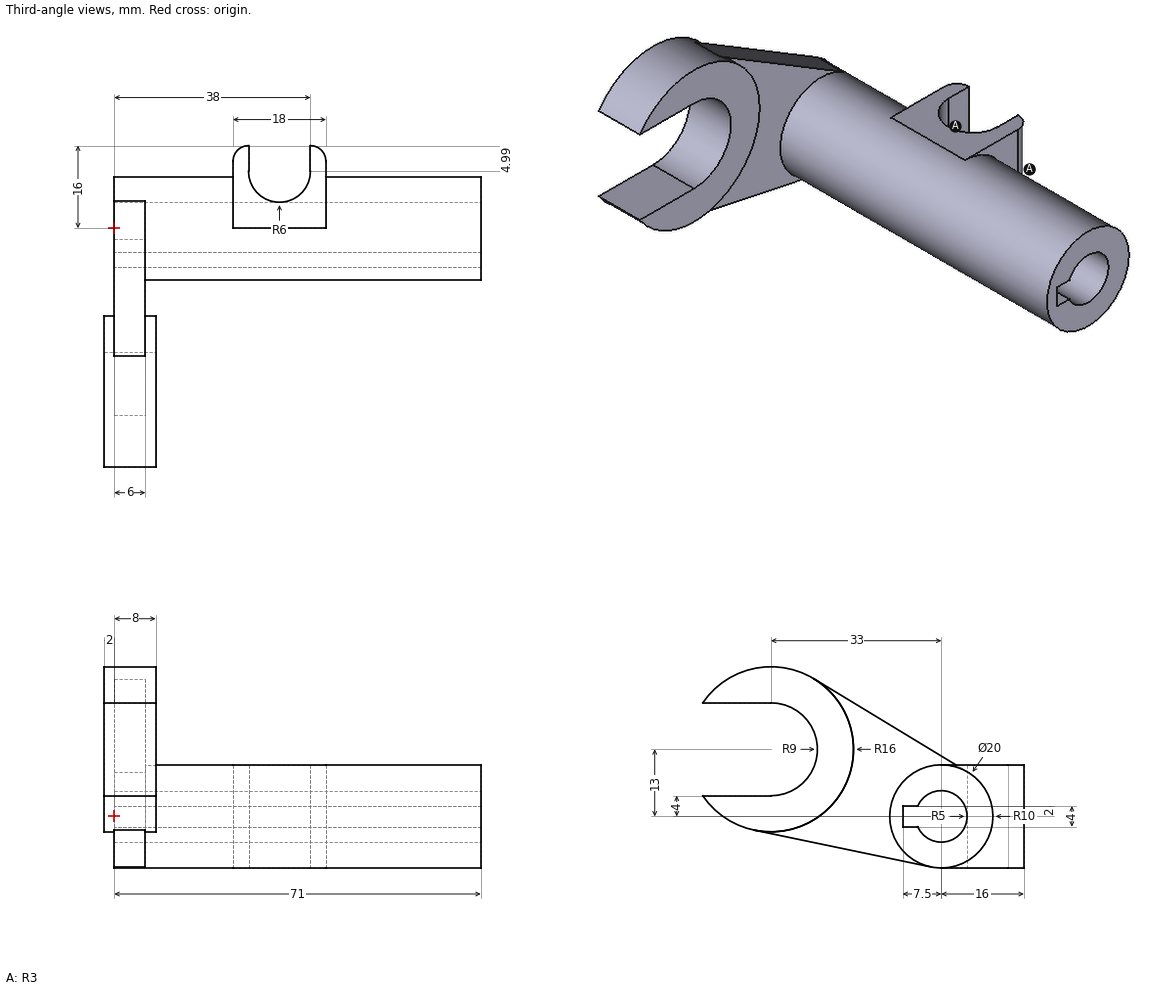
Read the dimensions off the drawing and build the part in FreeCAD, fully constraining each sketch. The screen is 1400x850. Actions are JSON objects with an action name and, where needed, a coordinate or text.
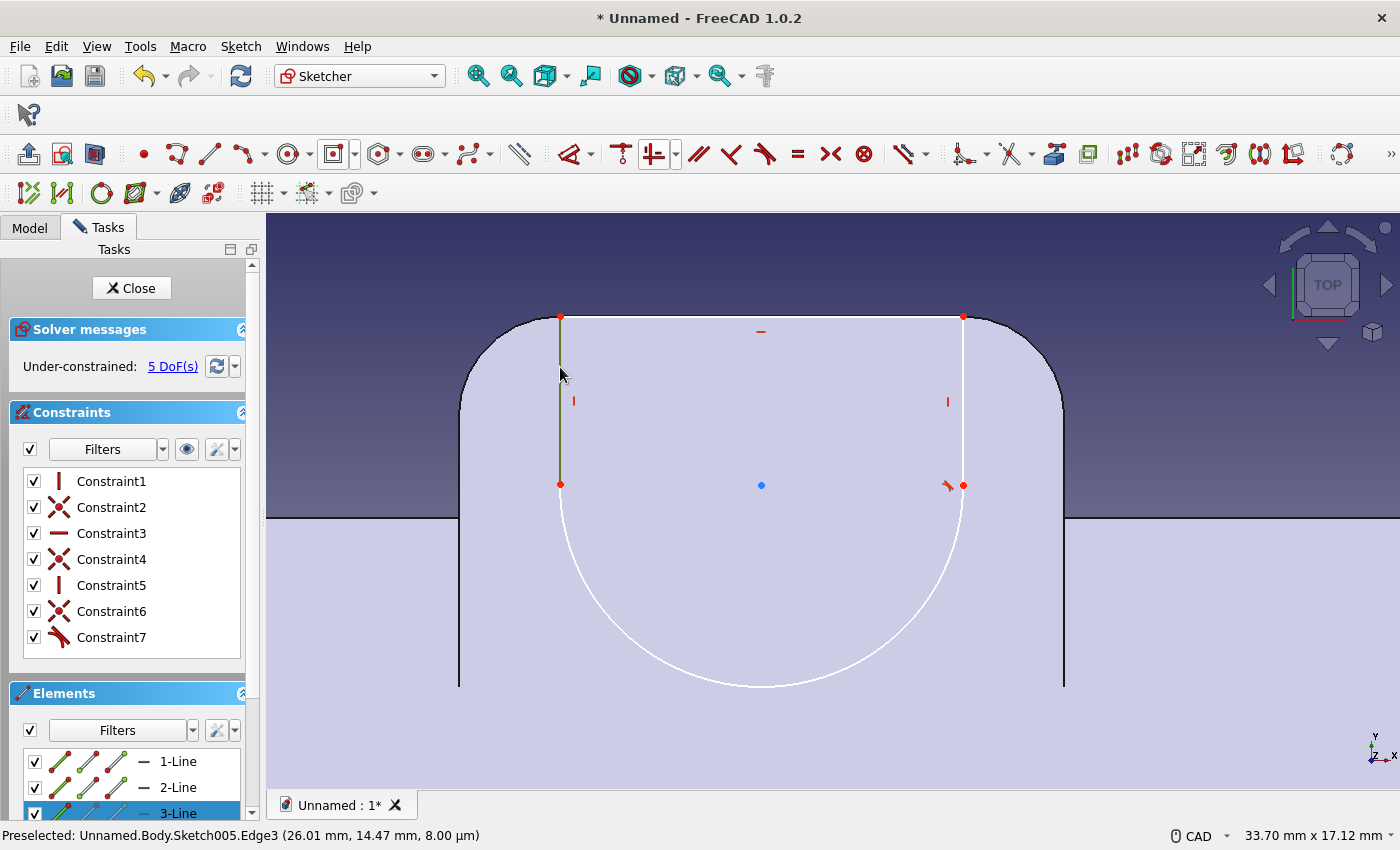
{"action": "left_click", "coordinate": [643, 648]}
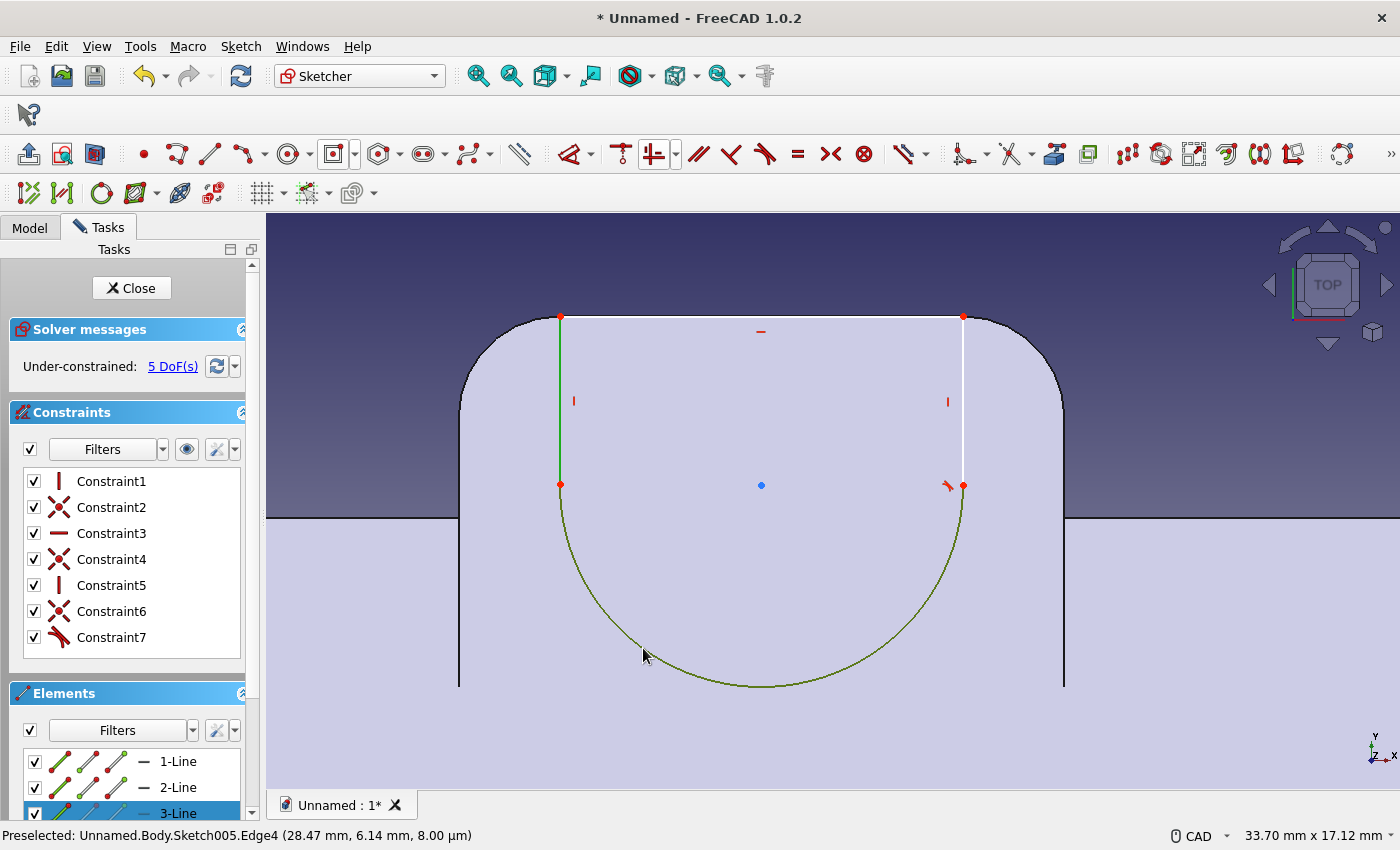
{"action": "key", "text": "t"}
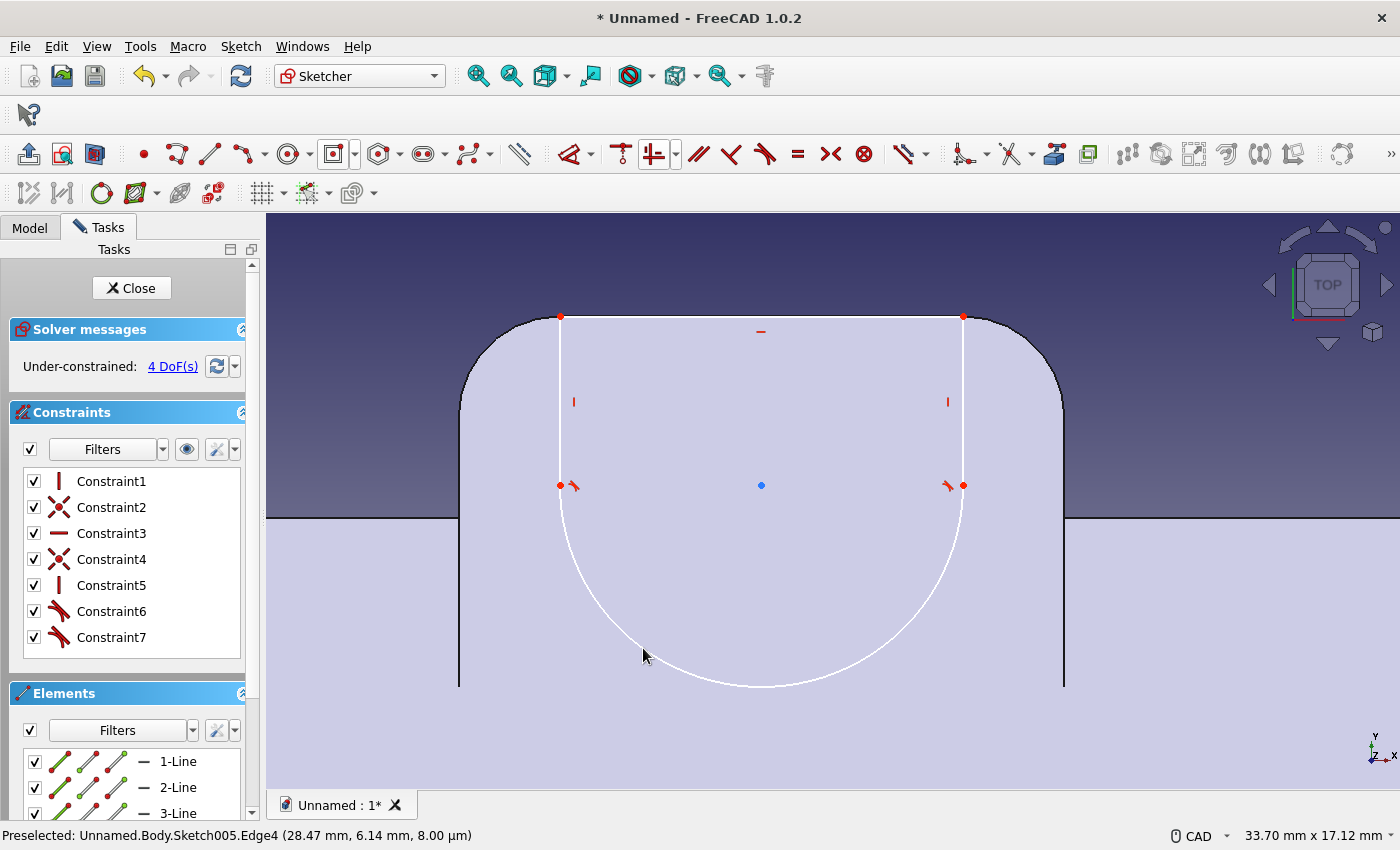
{"action": "left_click", "coordinate": [568, 154]}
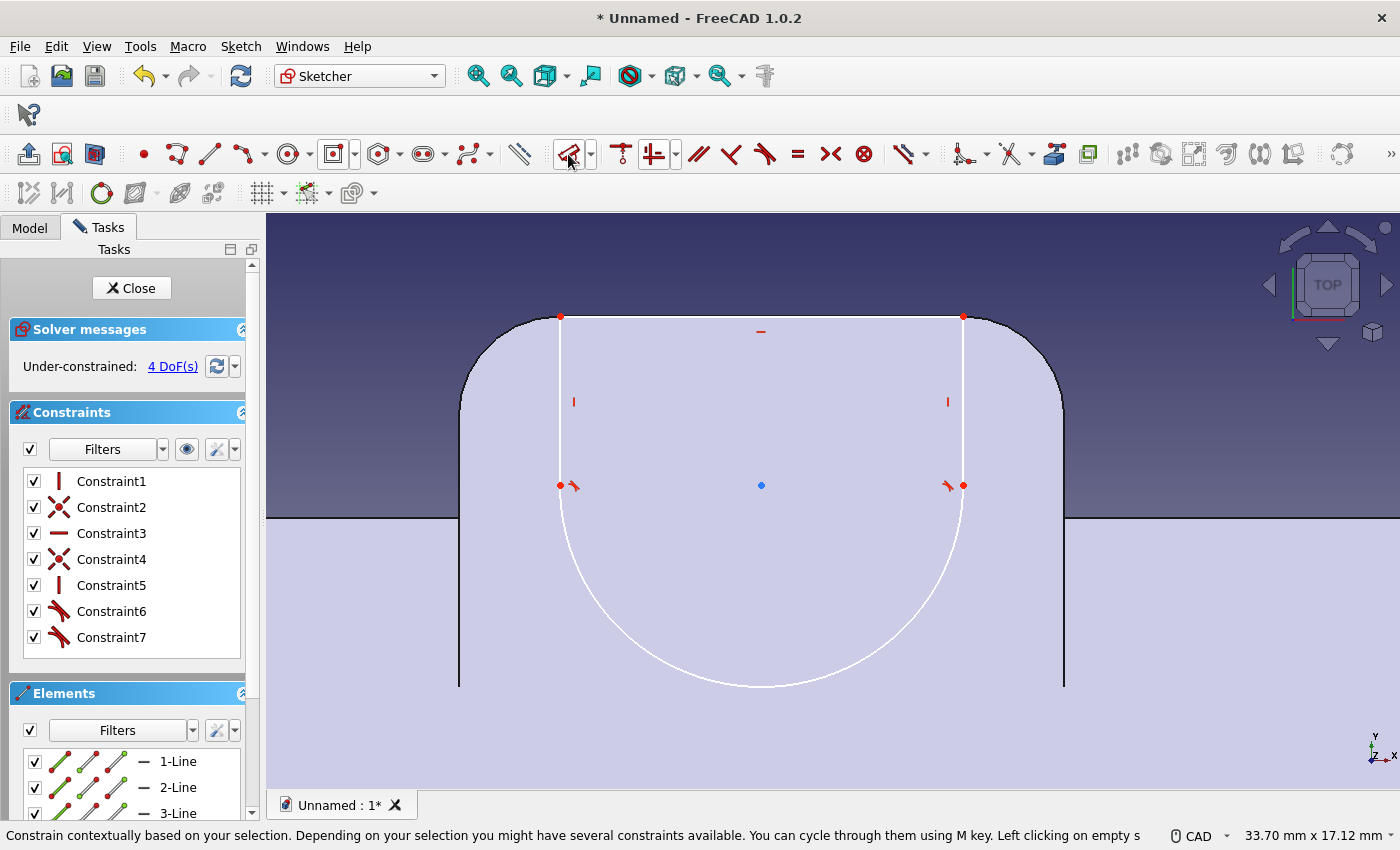
{"action": "left_click", "coordinate": [643, 649]}
{"action": "left_click", "coordinate": [624, 675]}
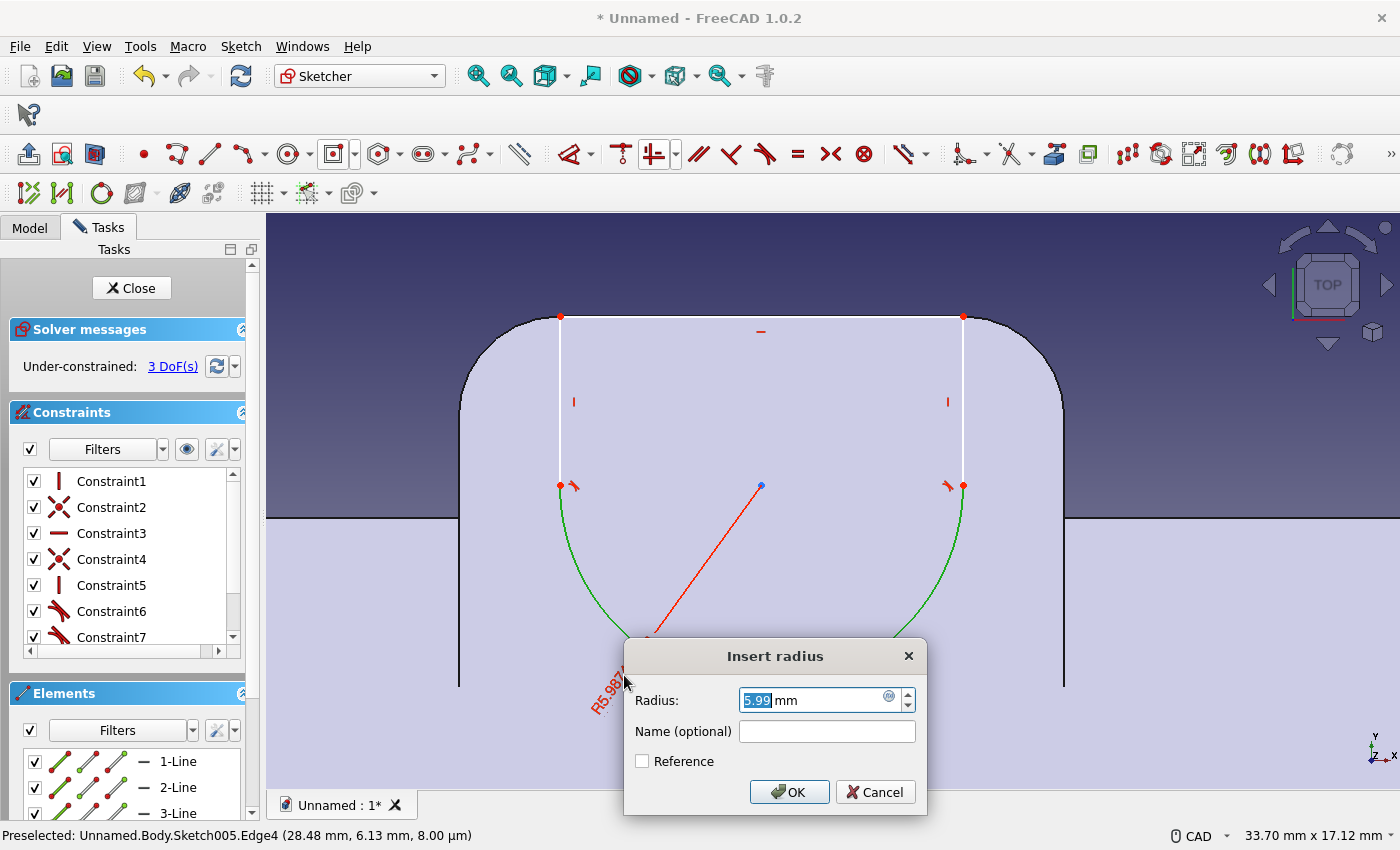
{"action": "type", "text": "6"}
{"action": "key", "text": "Return"}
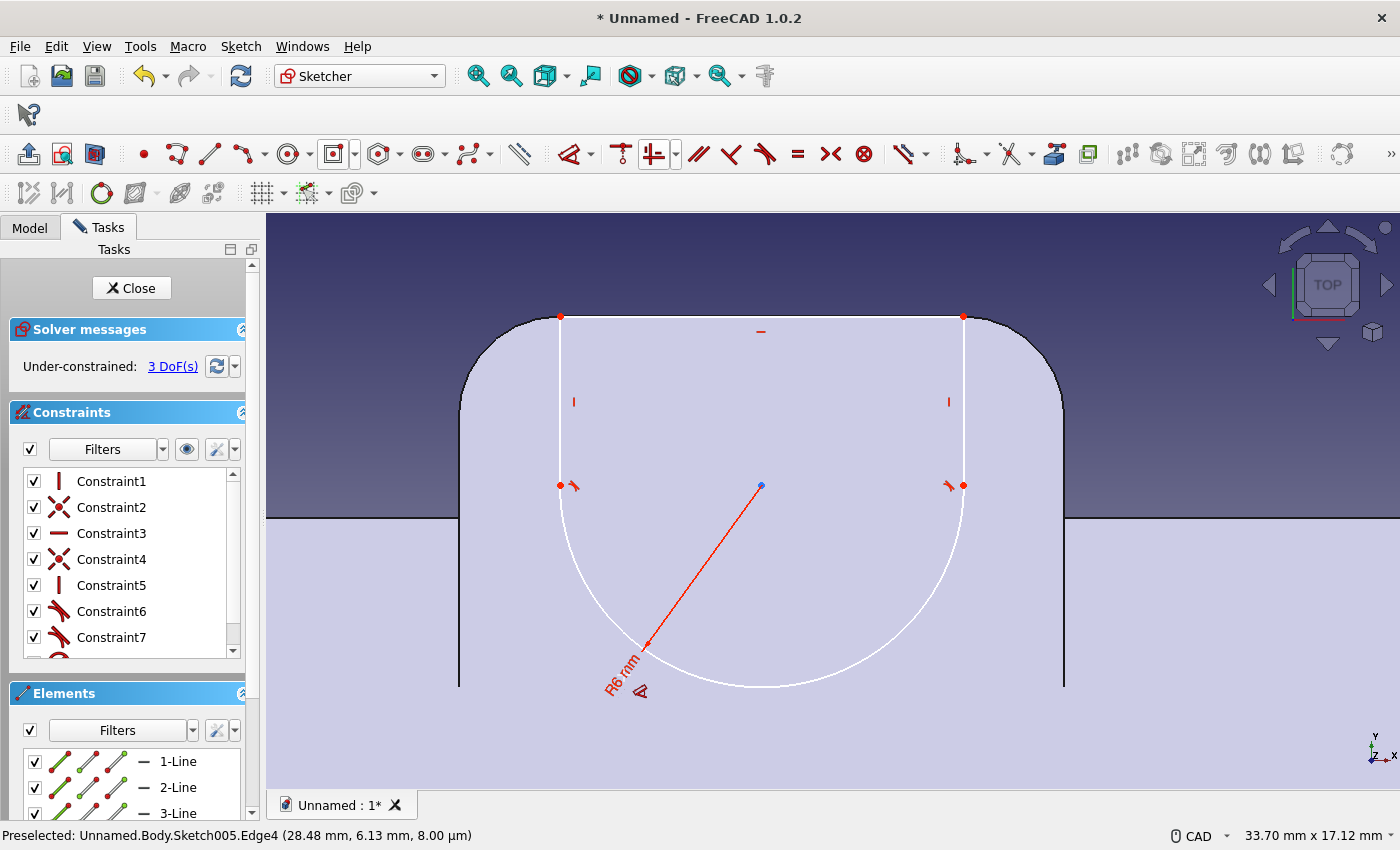
{"action": "left_click", "coordinate": [964, 486]}
{"action": "left_click", "coordinate": [629, 452]}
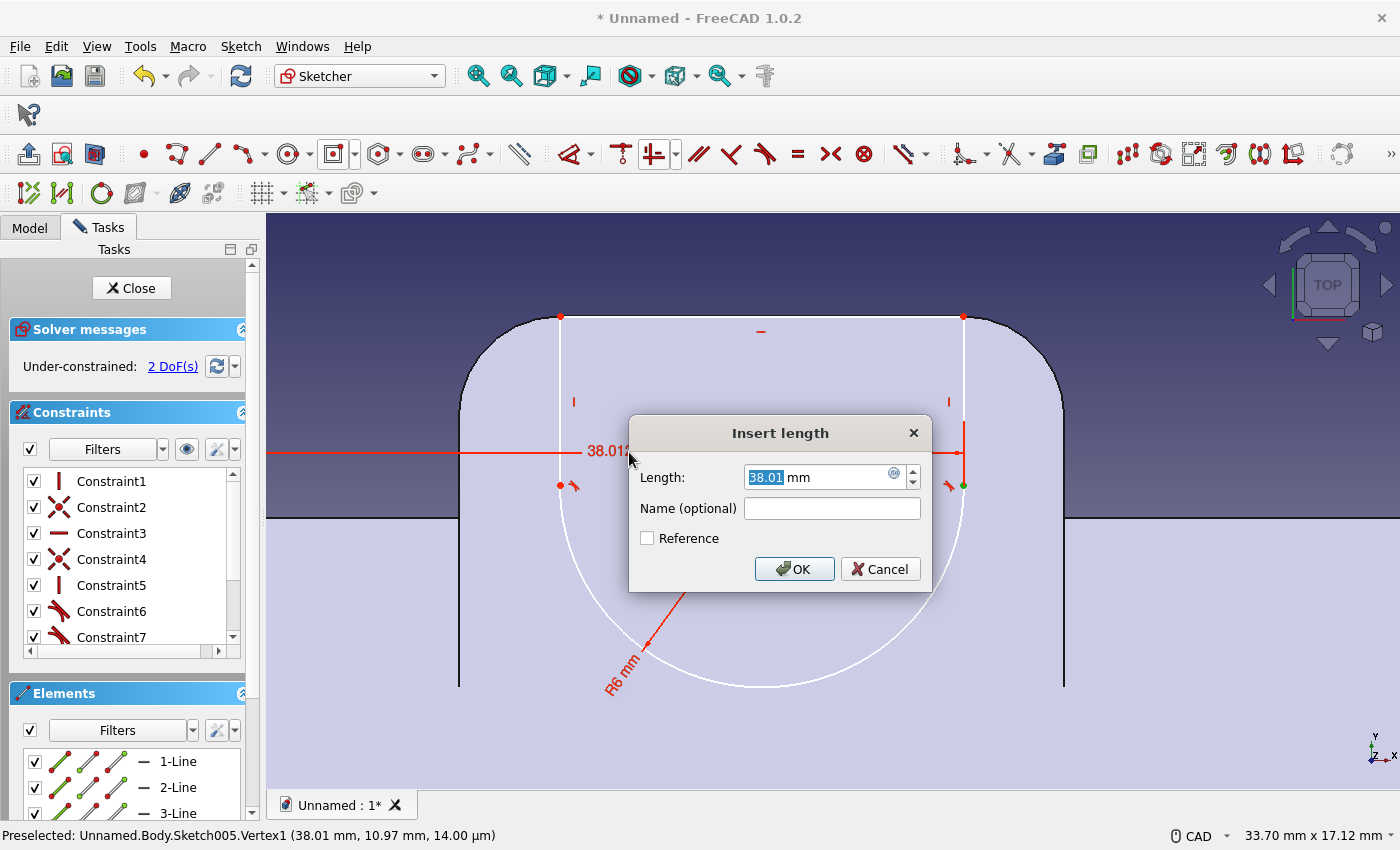
{"action": "type", "text": "38"}
{"action": "key", "text": "Return"}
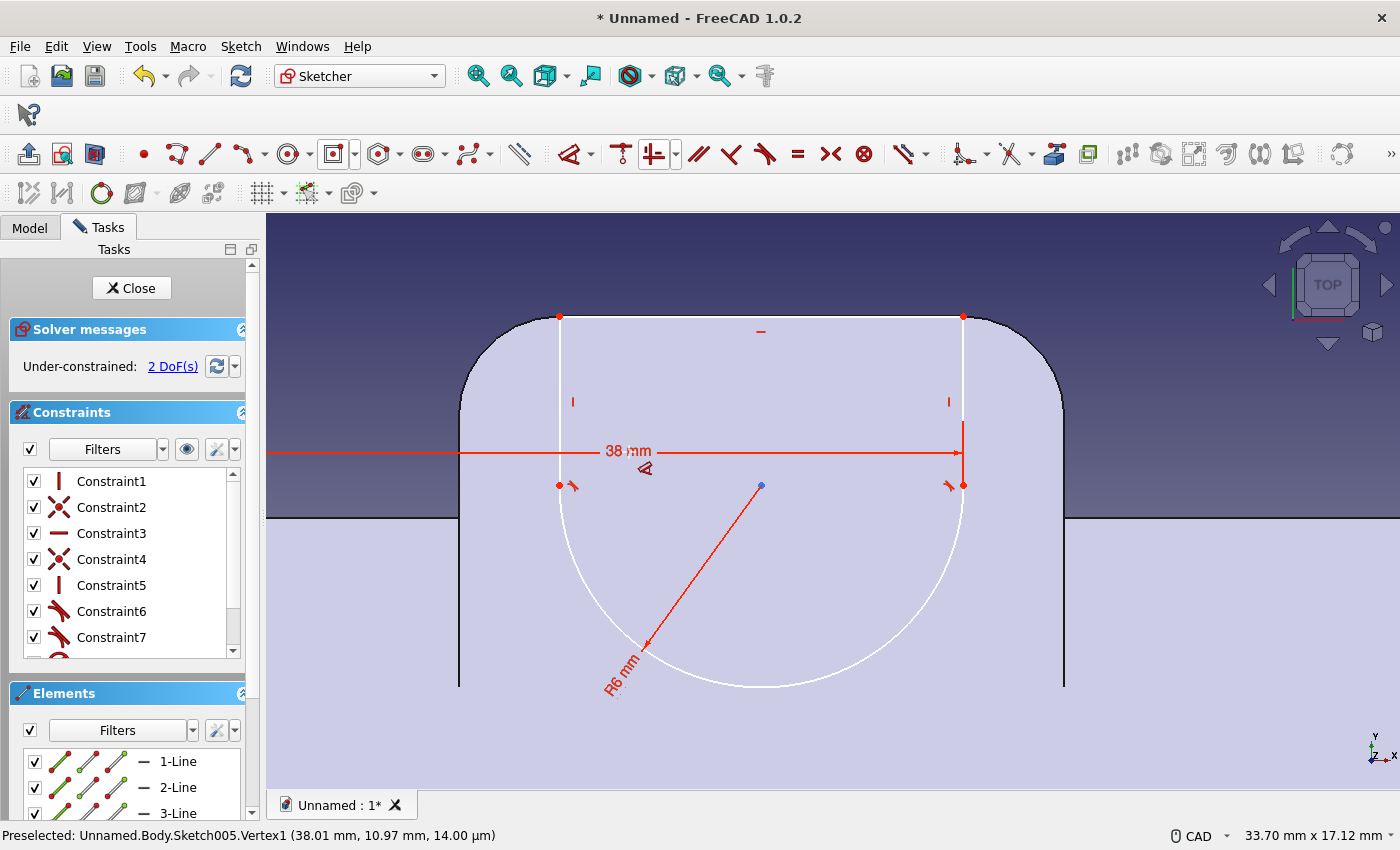
{"action": "left_click", "coordinate": [963, 317]}
{"action": "left_click", "coordinate": [997, 539]}